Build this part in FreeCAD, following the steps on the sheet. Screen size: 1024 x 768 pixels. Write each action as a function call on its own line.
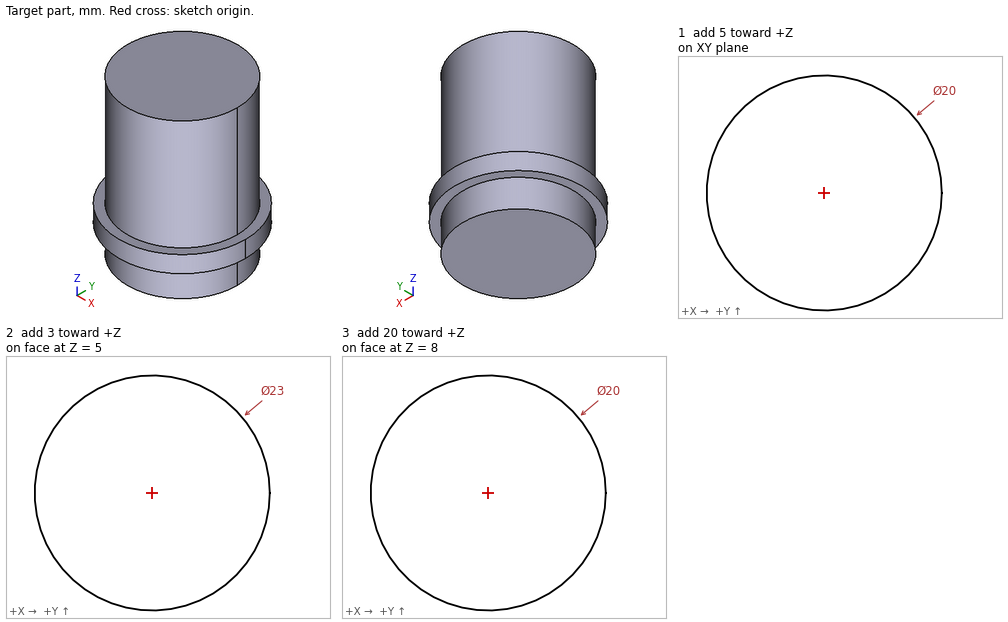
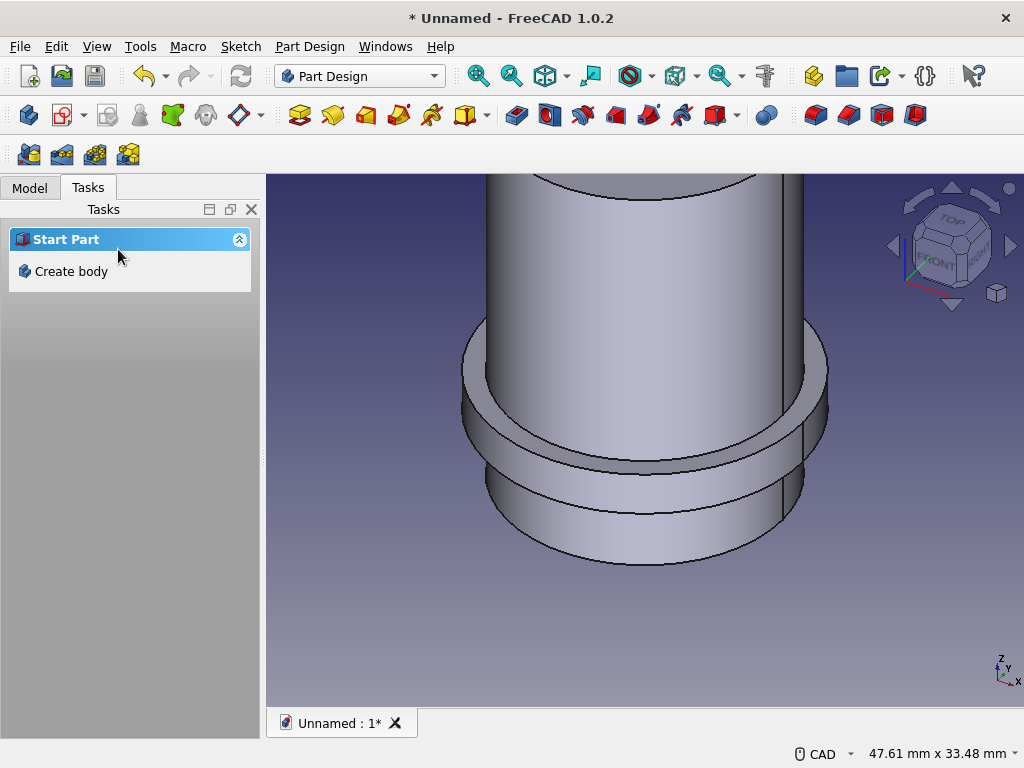
key(0)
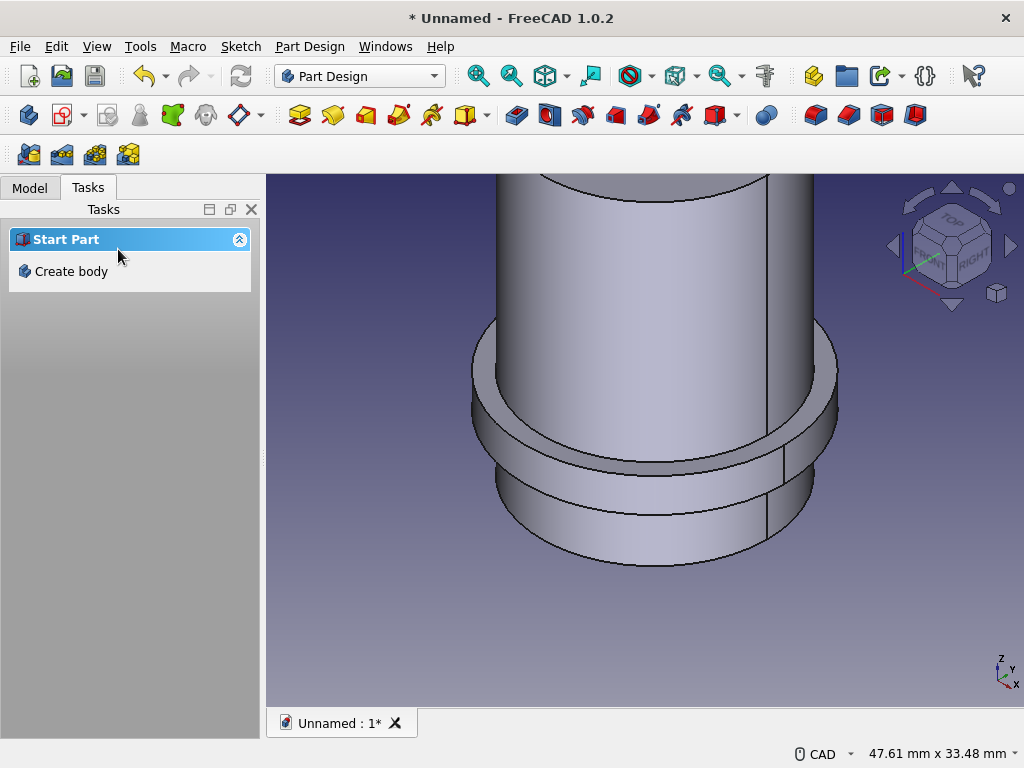
click(479, 76)